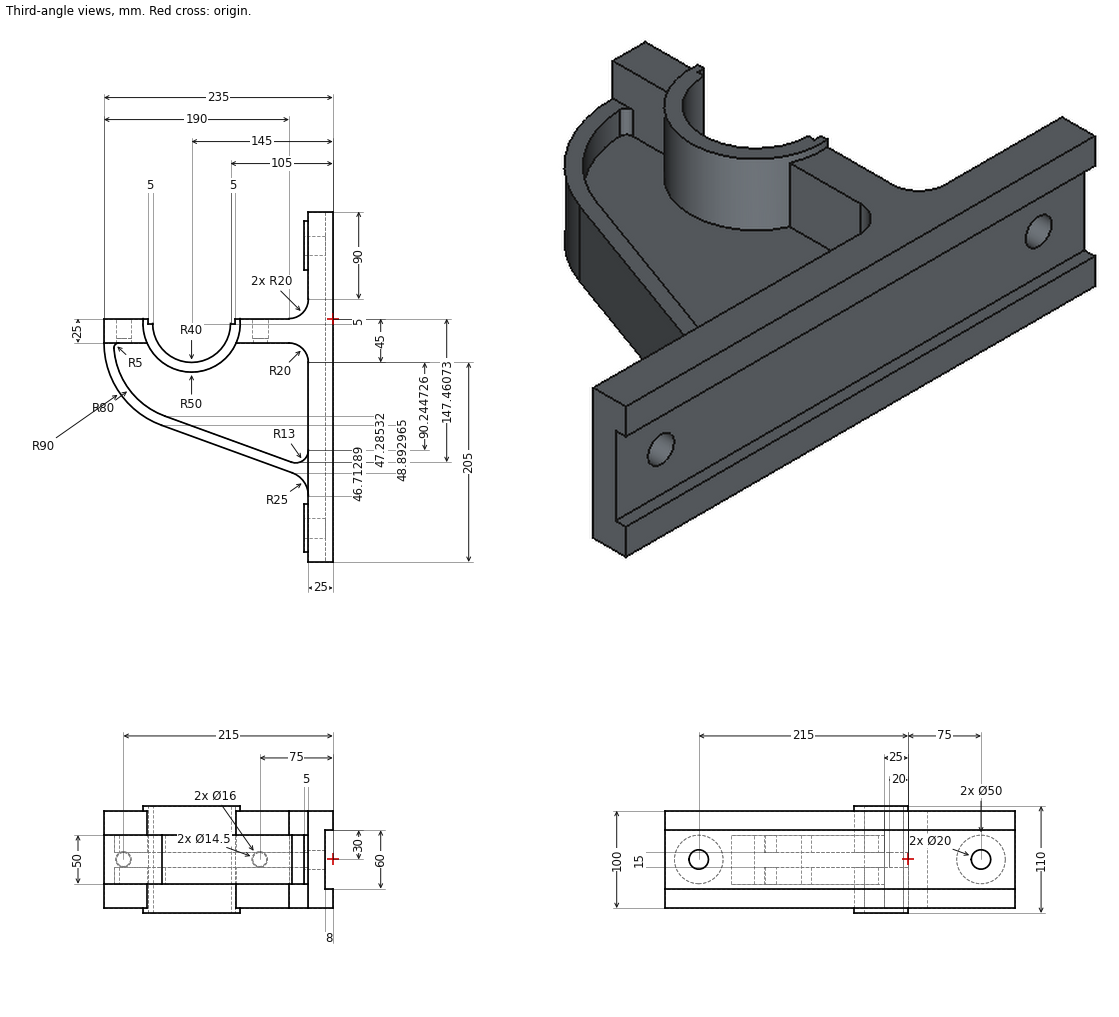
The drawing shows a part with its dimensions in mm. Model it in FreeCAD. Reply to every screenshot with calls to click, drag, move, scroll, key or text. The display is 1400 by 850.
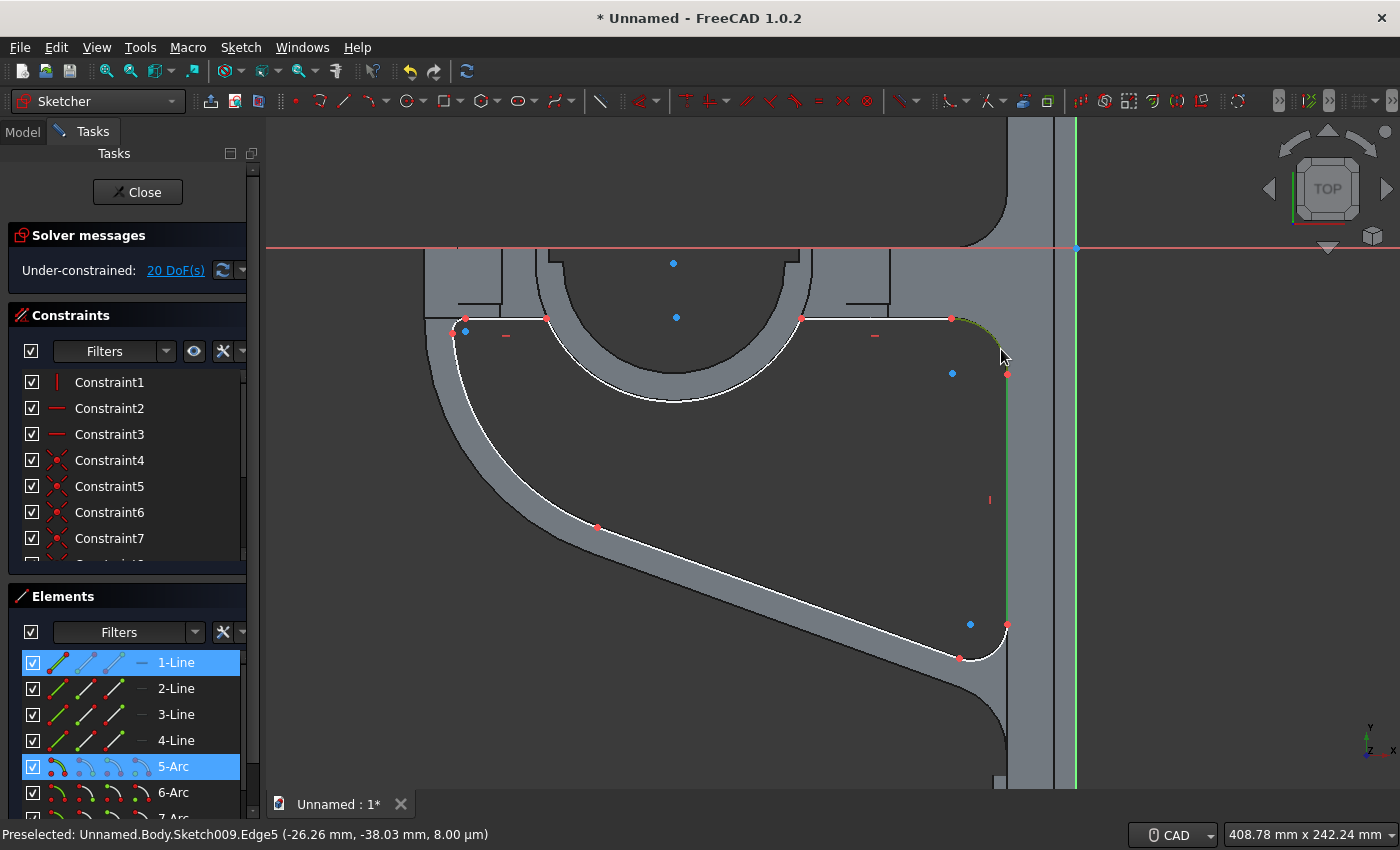
click(796, 102)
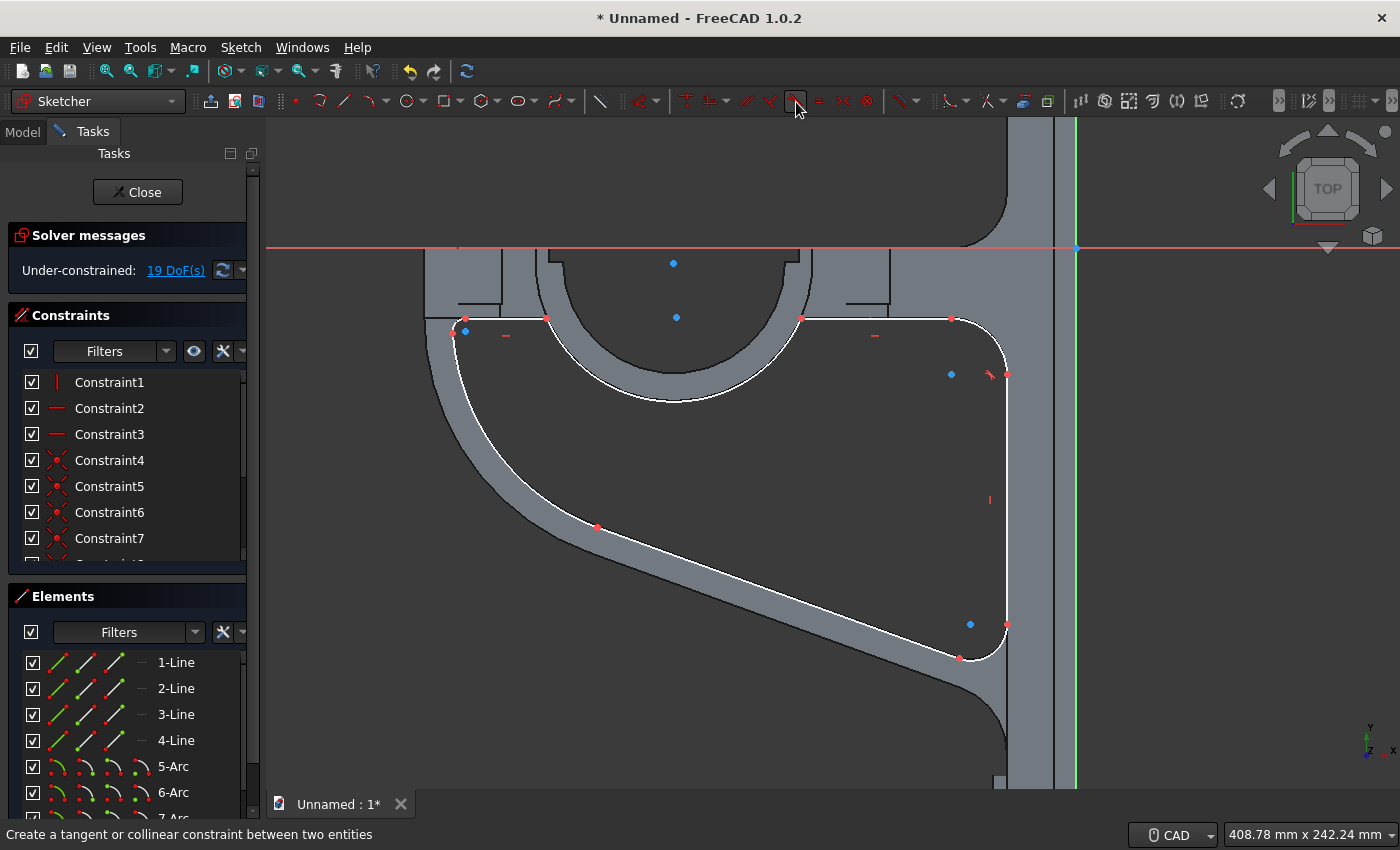
click(1007, 550)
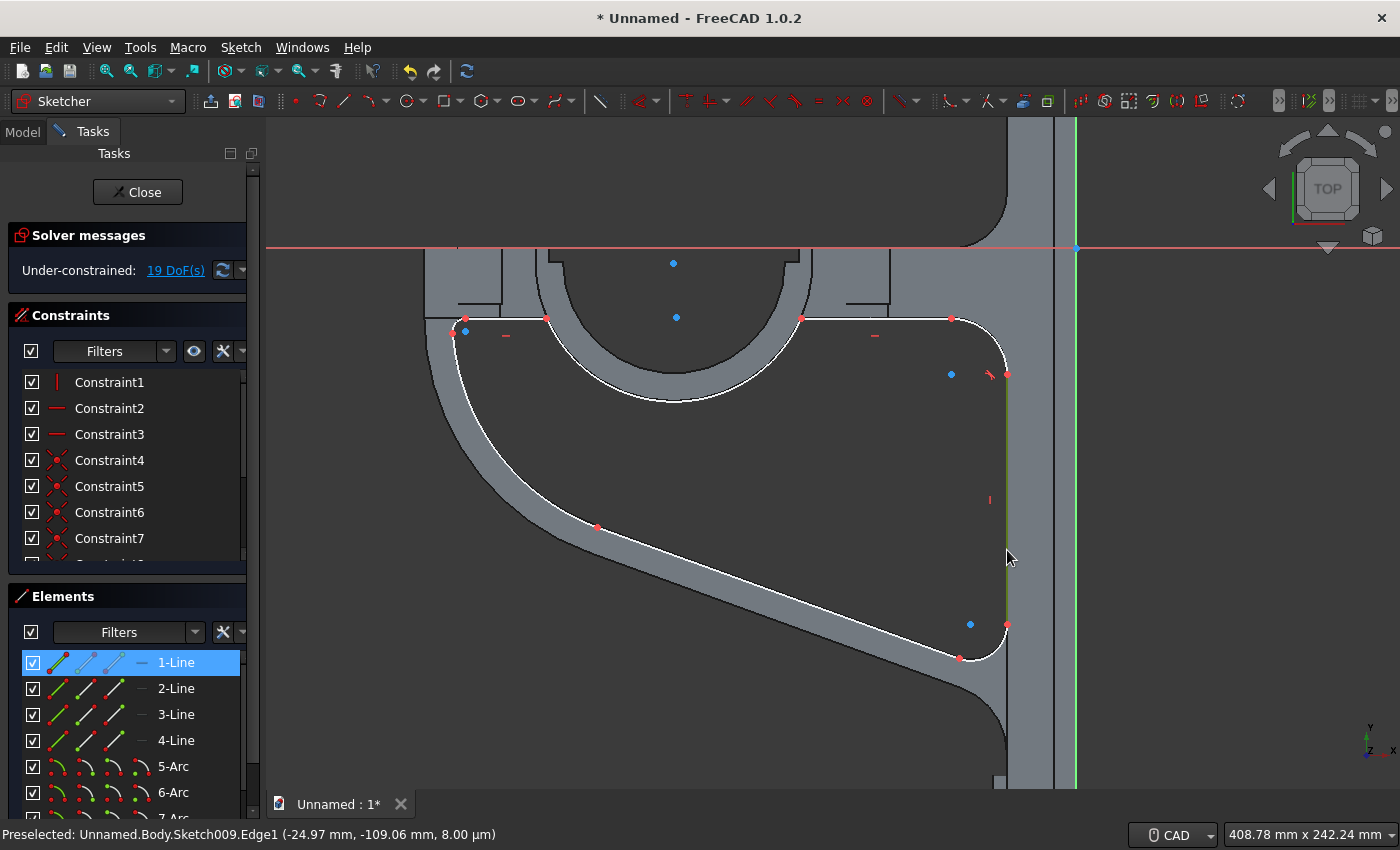
click(979, 660)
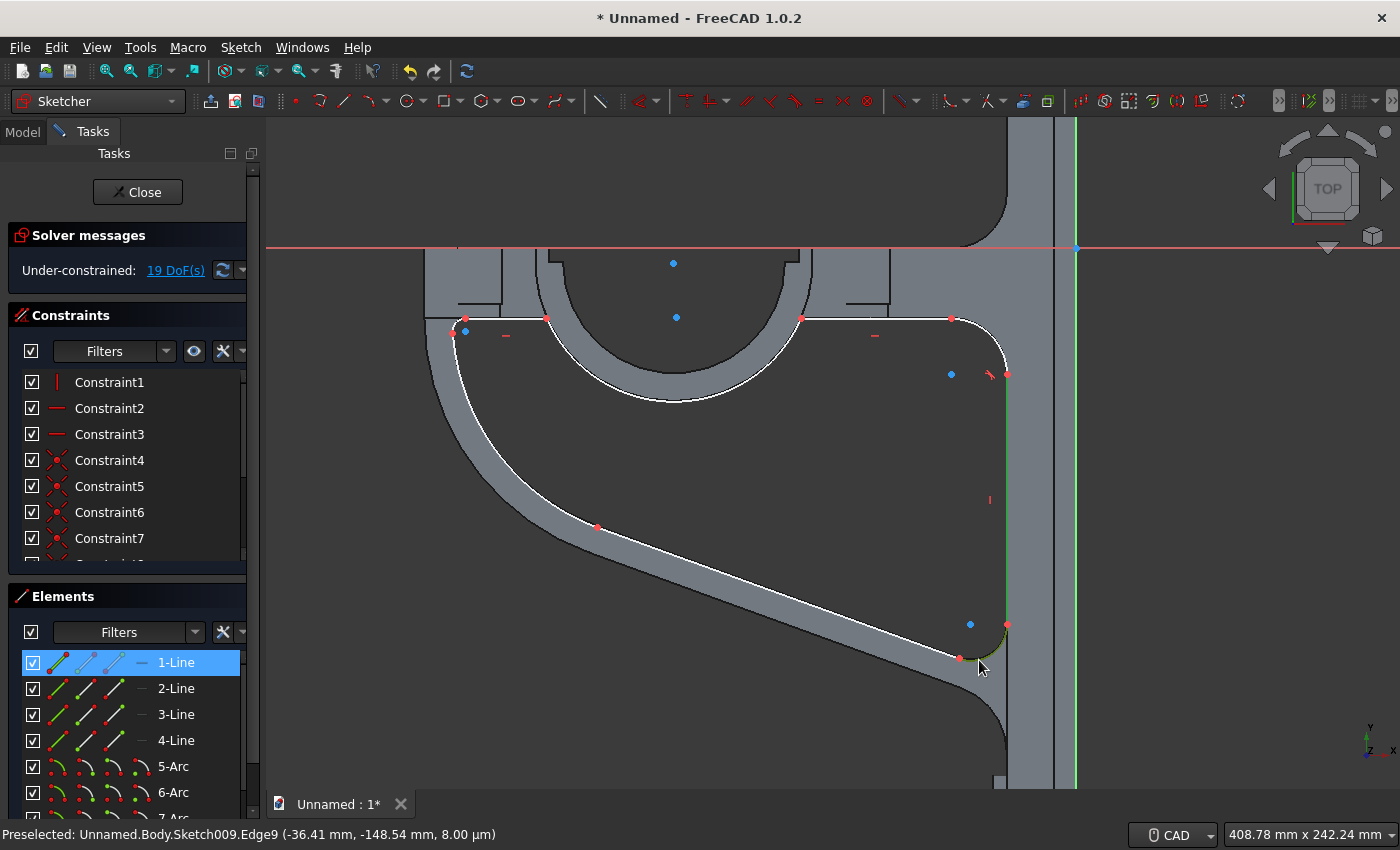
click(796, 102)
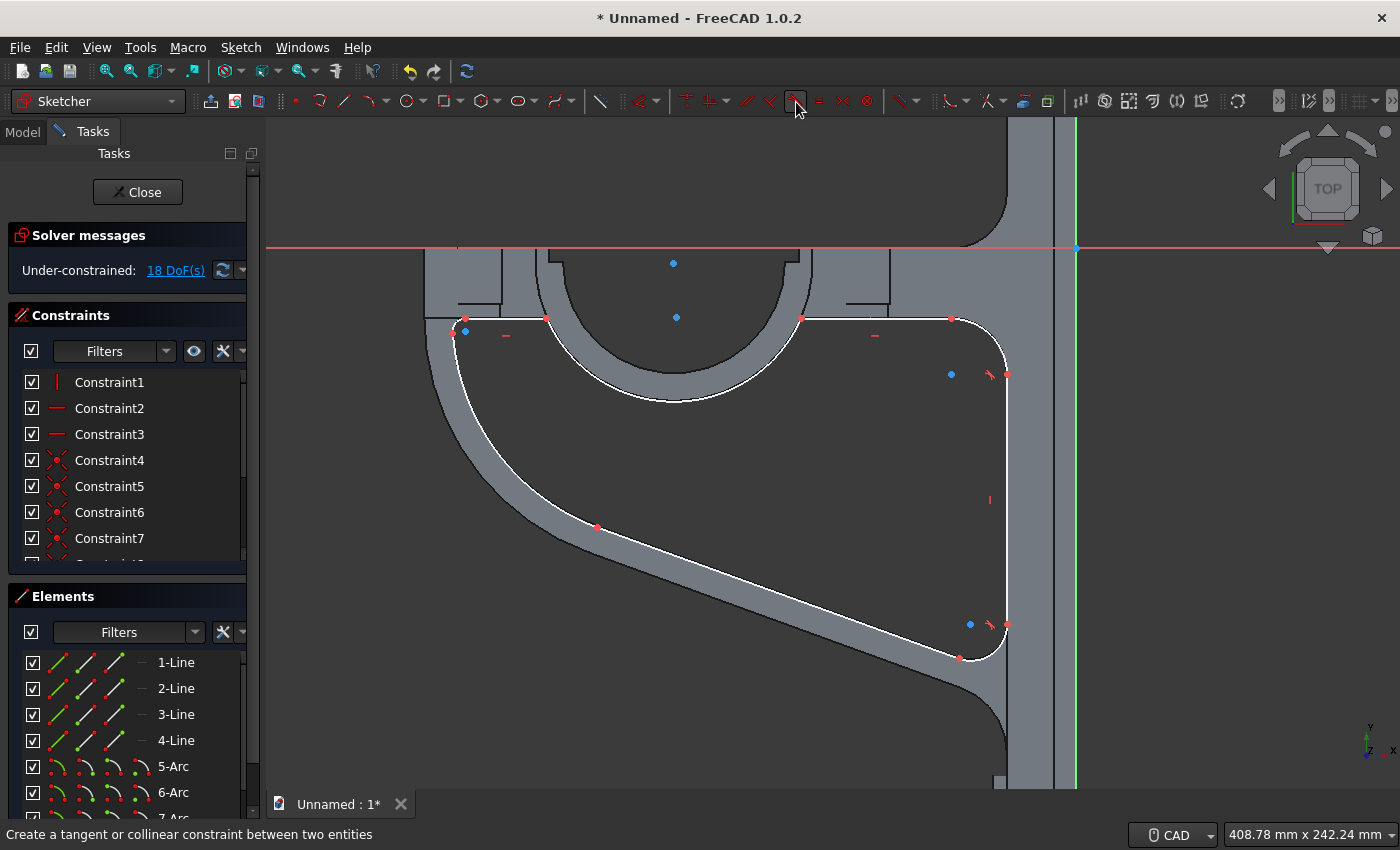
click(906, 319)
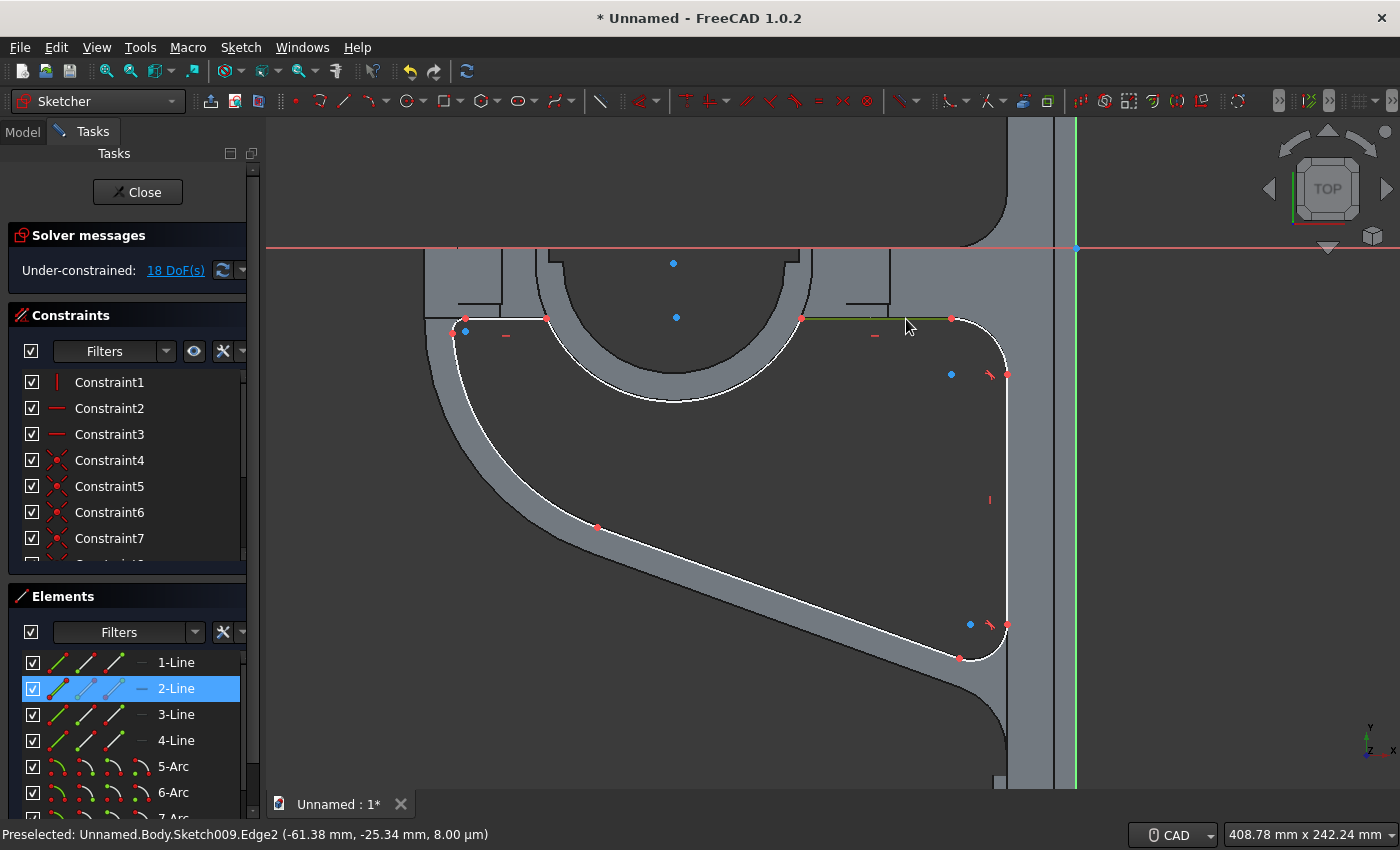
click(1001, 349)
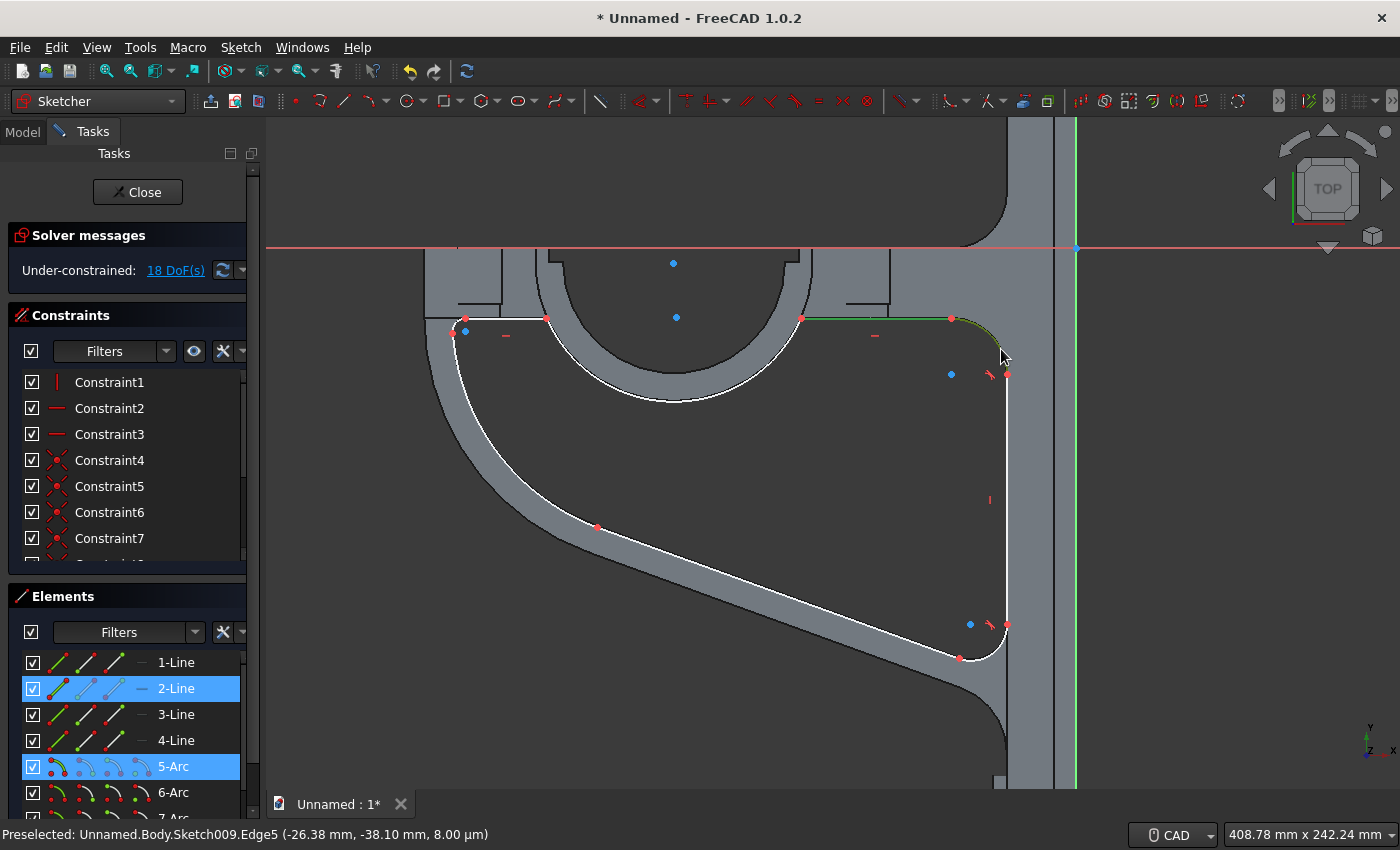
click(796, 102)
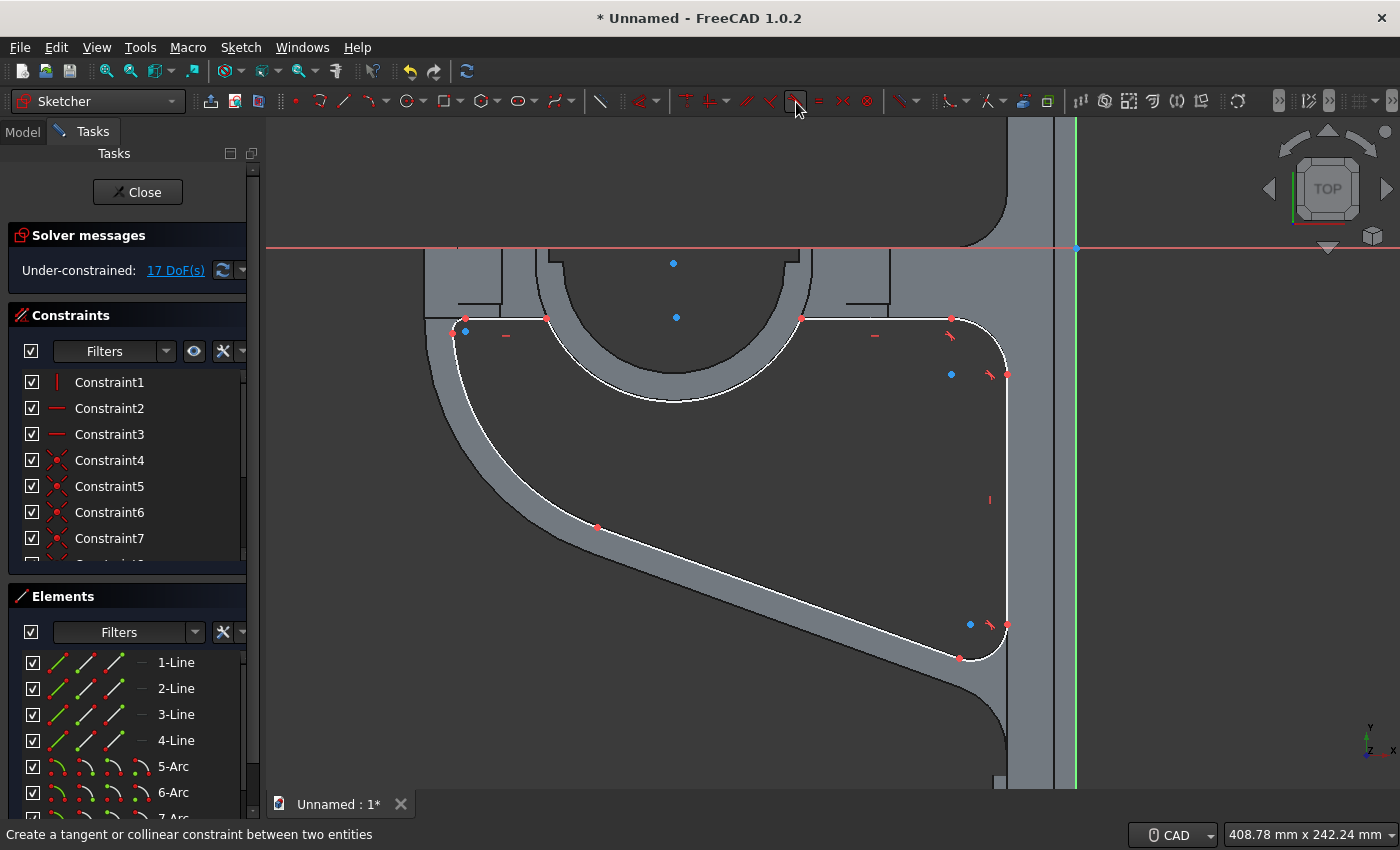
click(523, 319)